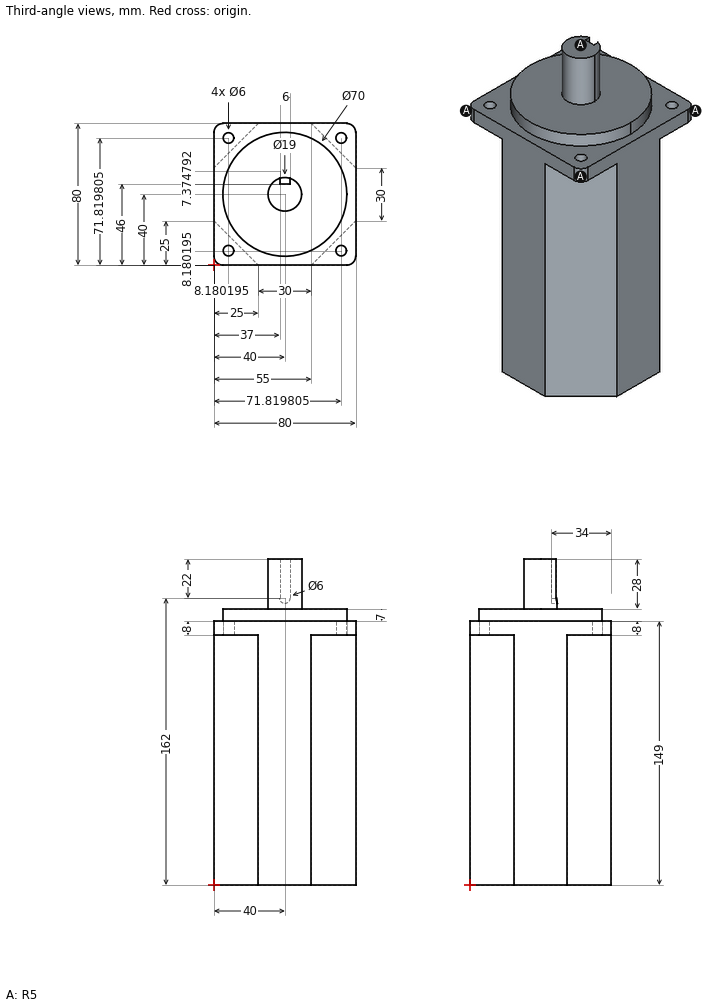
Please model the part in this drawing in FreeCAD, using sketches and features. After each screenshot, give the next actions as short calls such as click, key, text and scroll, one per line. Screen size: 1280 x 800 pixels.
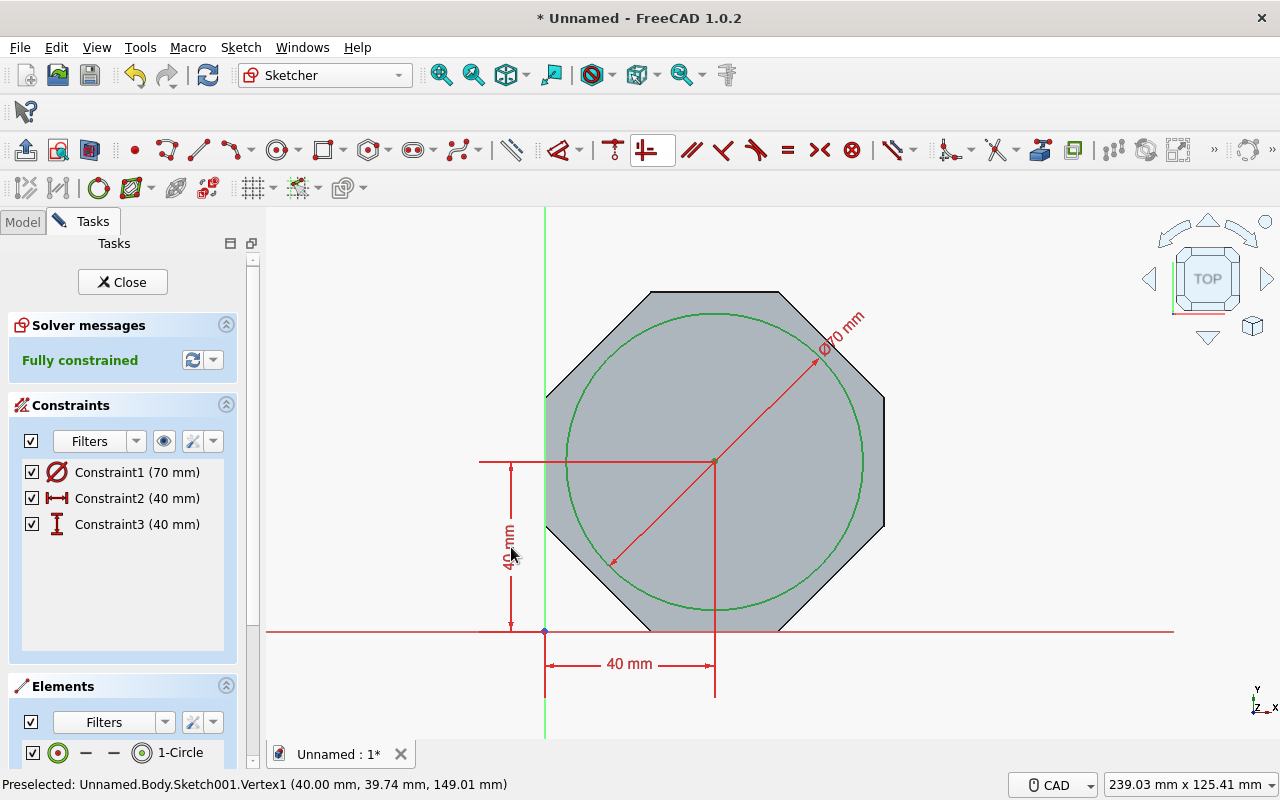
click(123, 282)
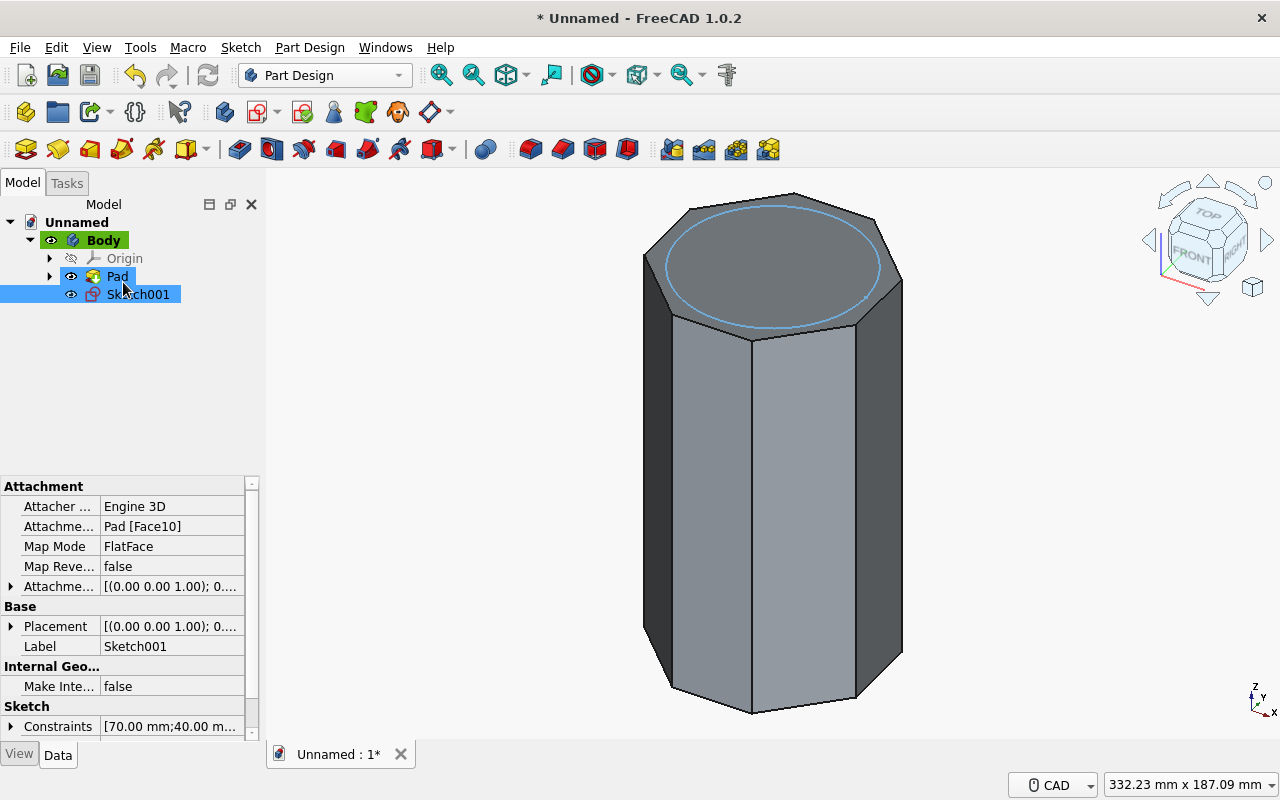
click(26, 150)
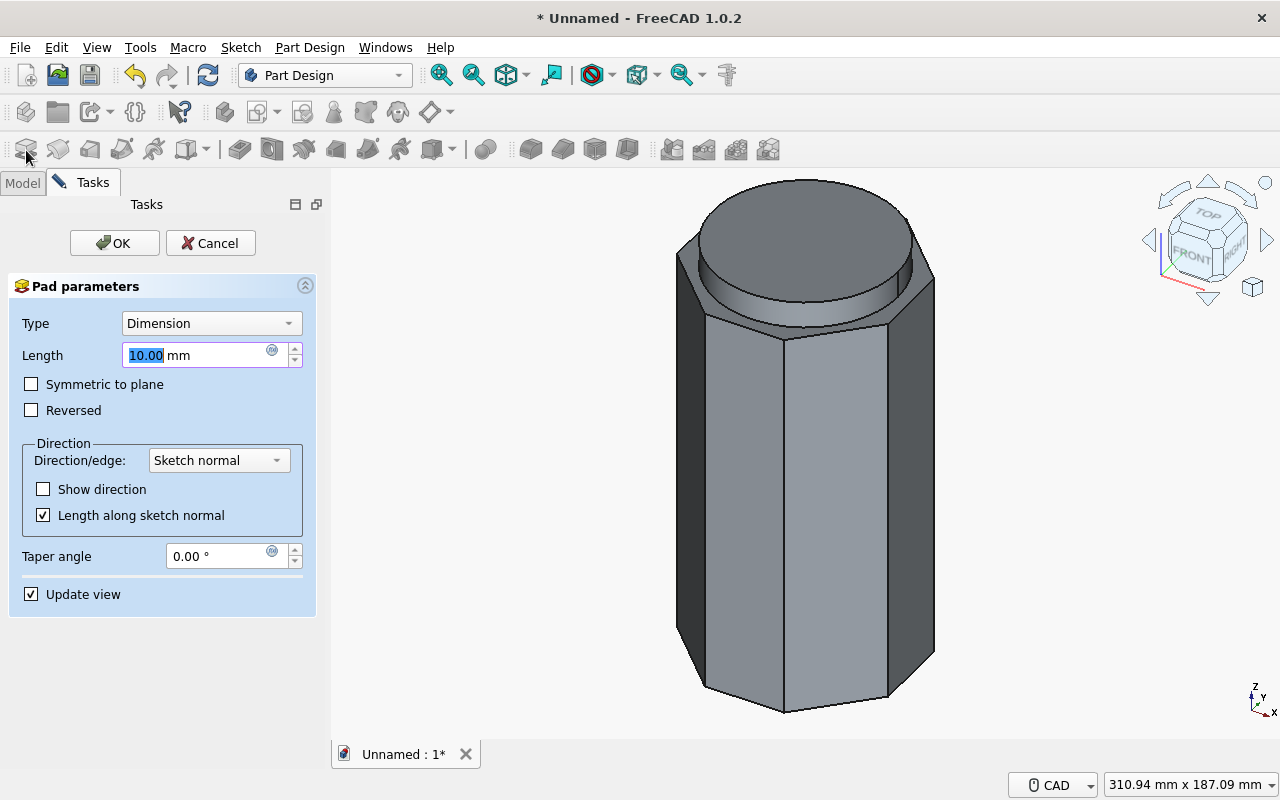
text(7)
key(Tab)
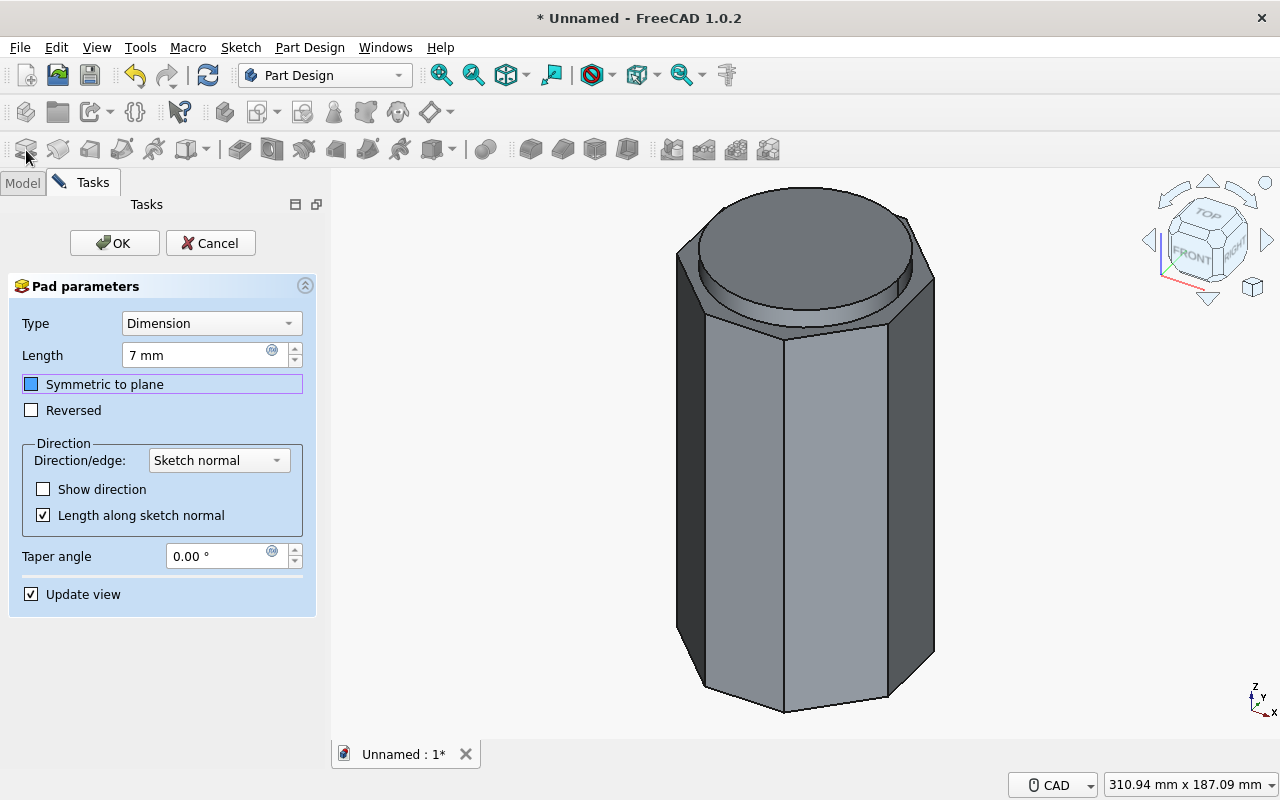
click(115, 243)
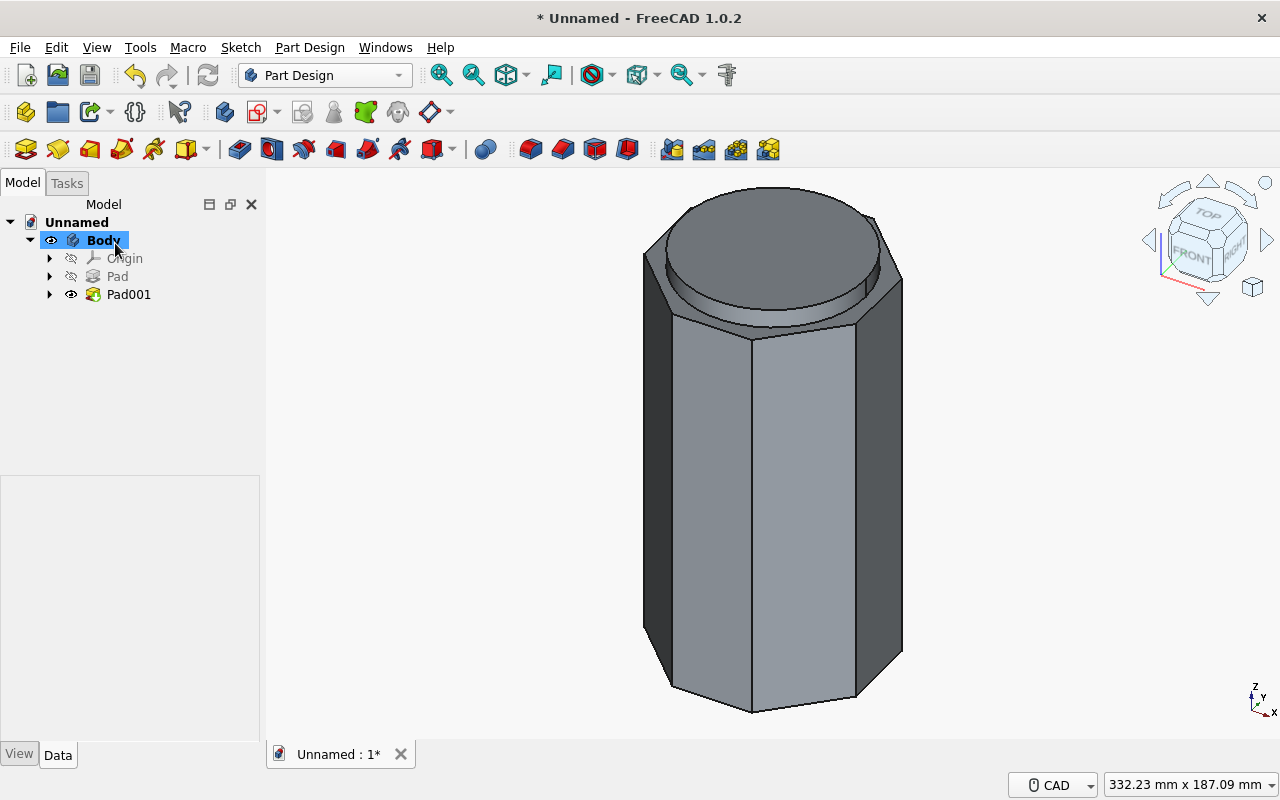
click(442, 76)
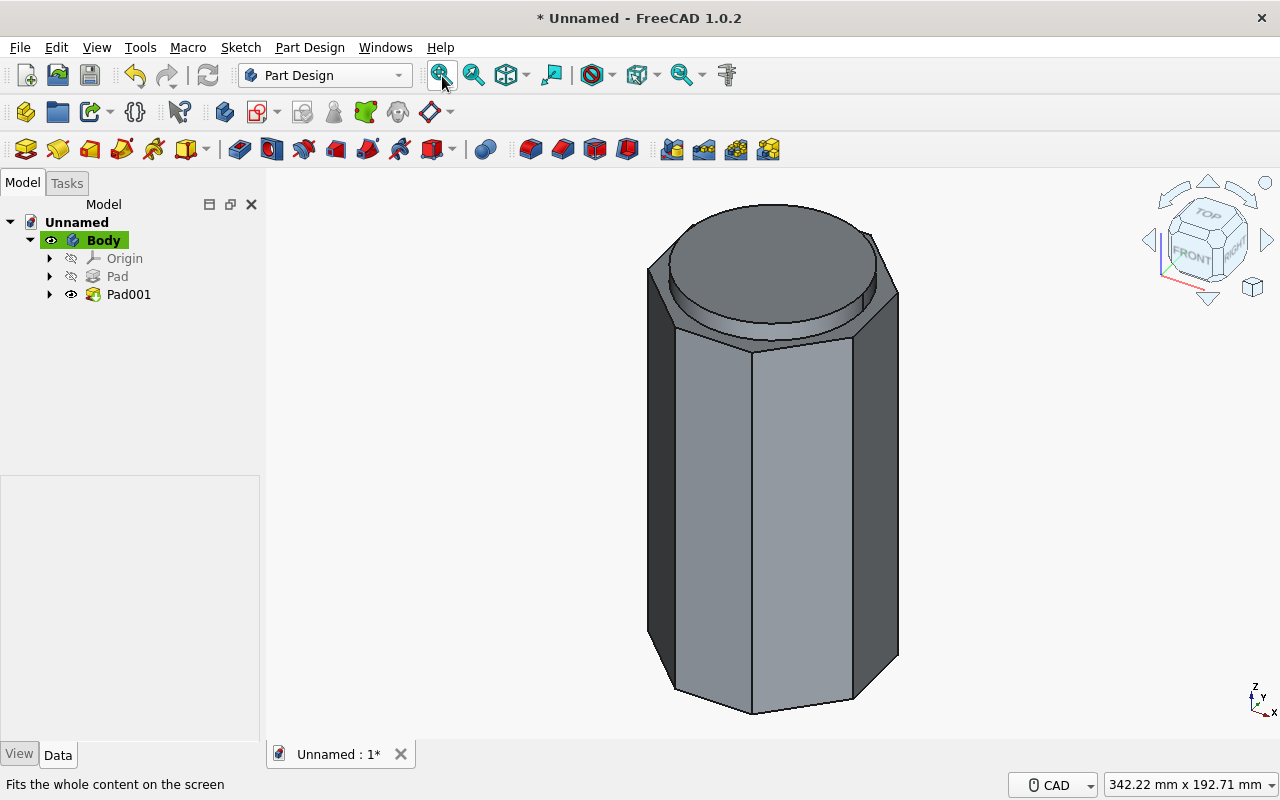
scroll(878, 292, up, 7)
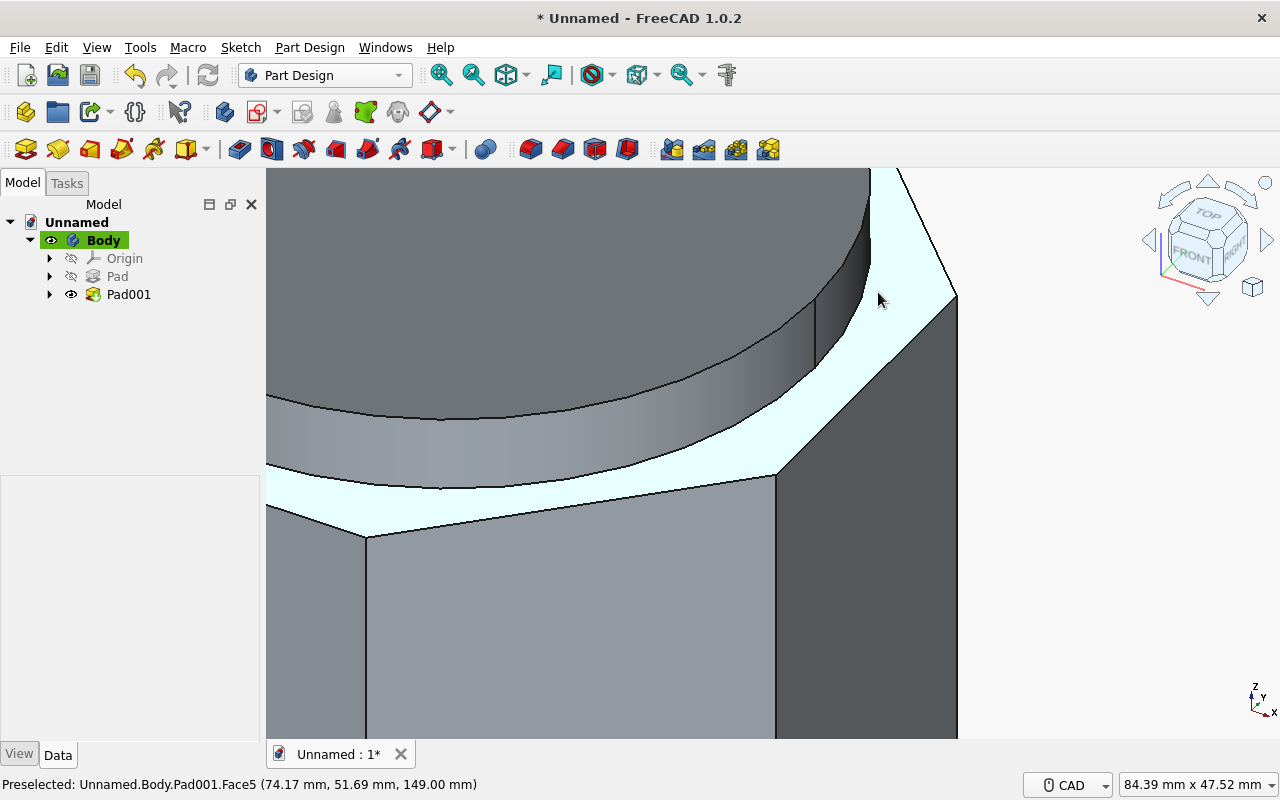
click(876, 296)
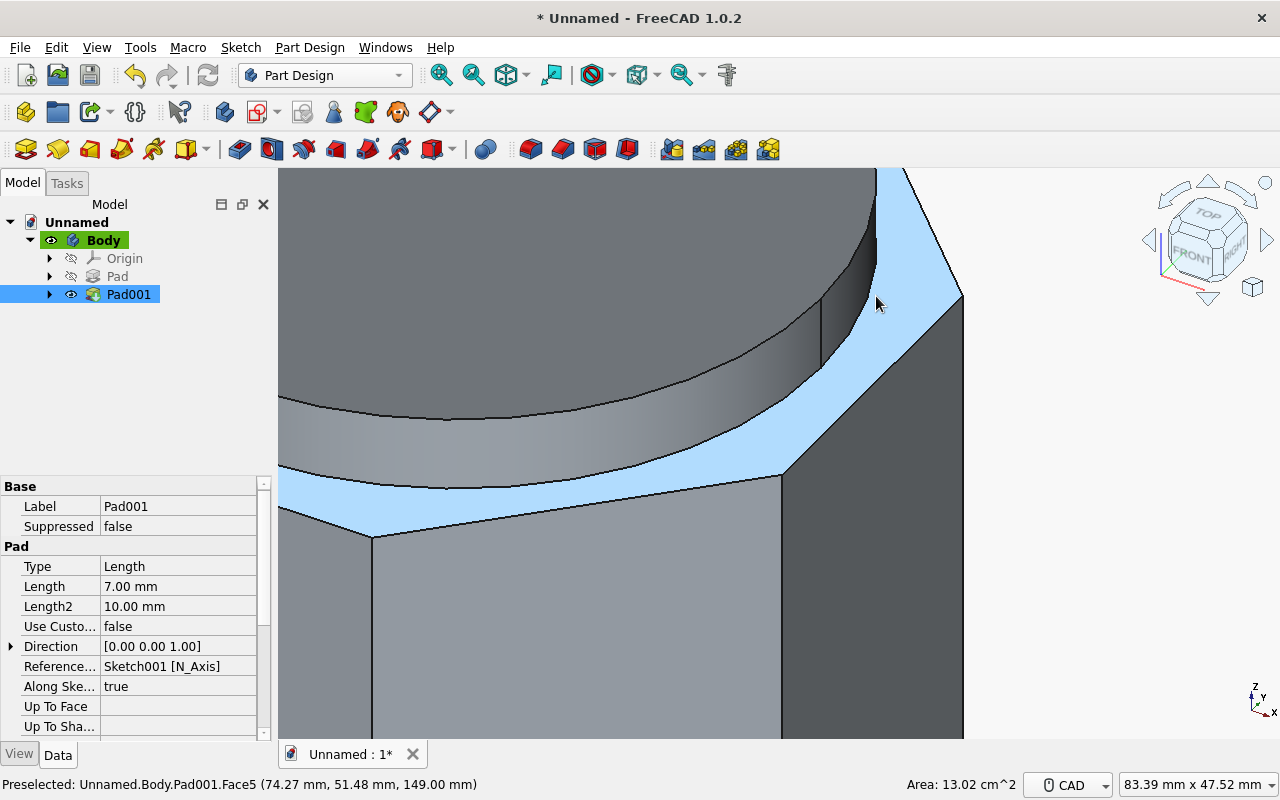
click(258, 112)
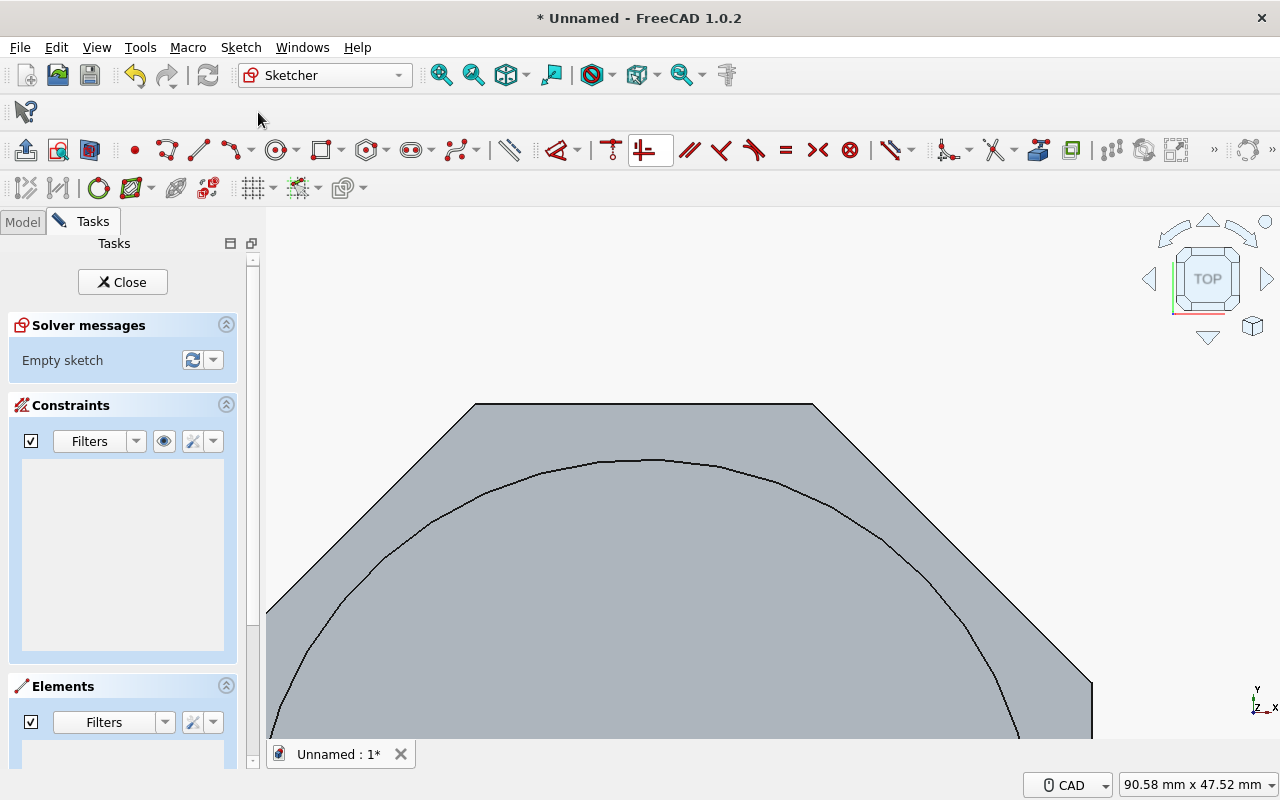
key(q)
key(s)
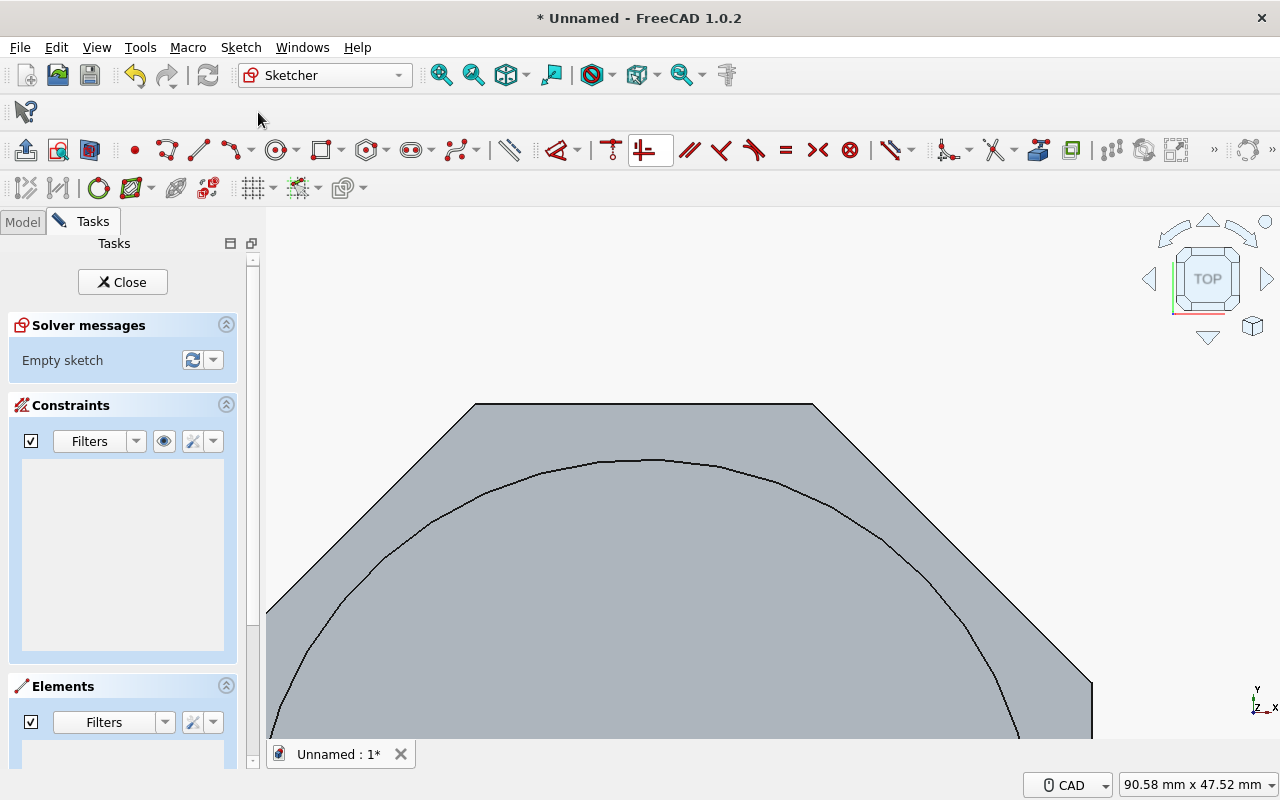
scroll(740, 253, down, 5)